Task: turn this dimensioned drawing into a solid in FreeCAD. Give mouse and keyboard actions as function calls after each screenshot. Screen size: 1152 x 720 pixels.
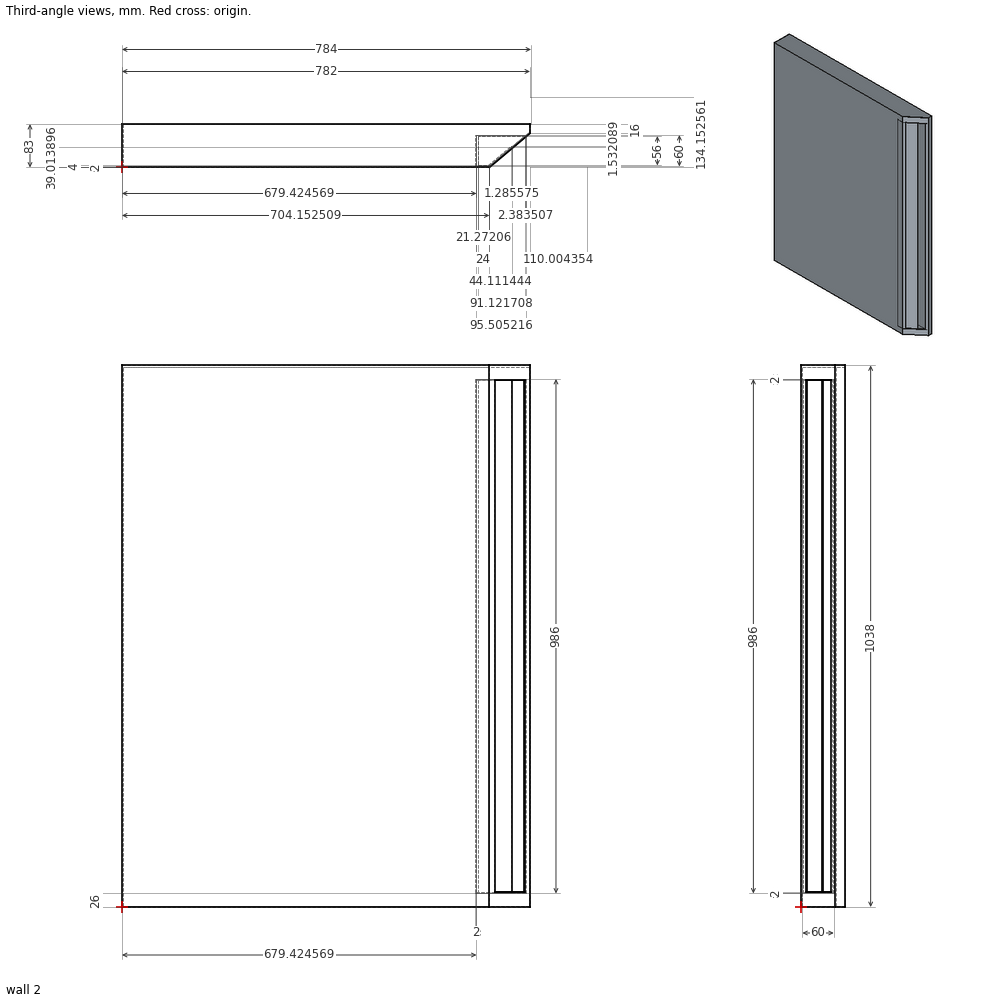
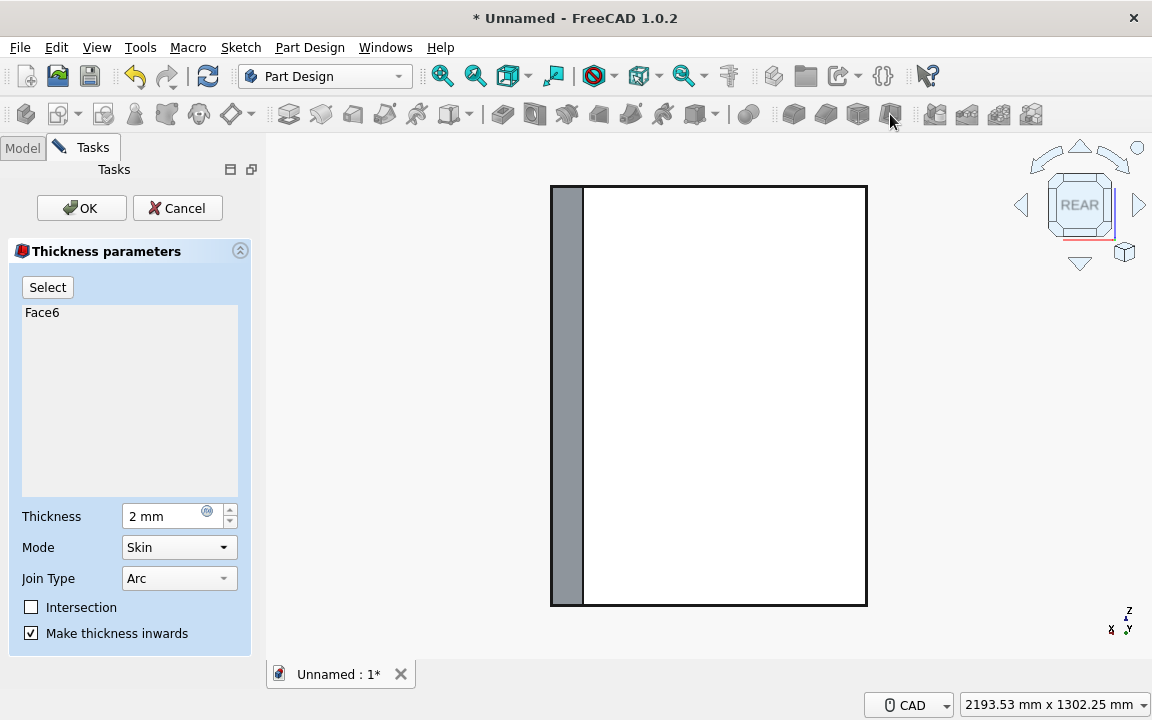
click(180, 578)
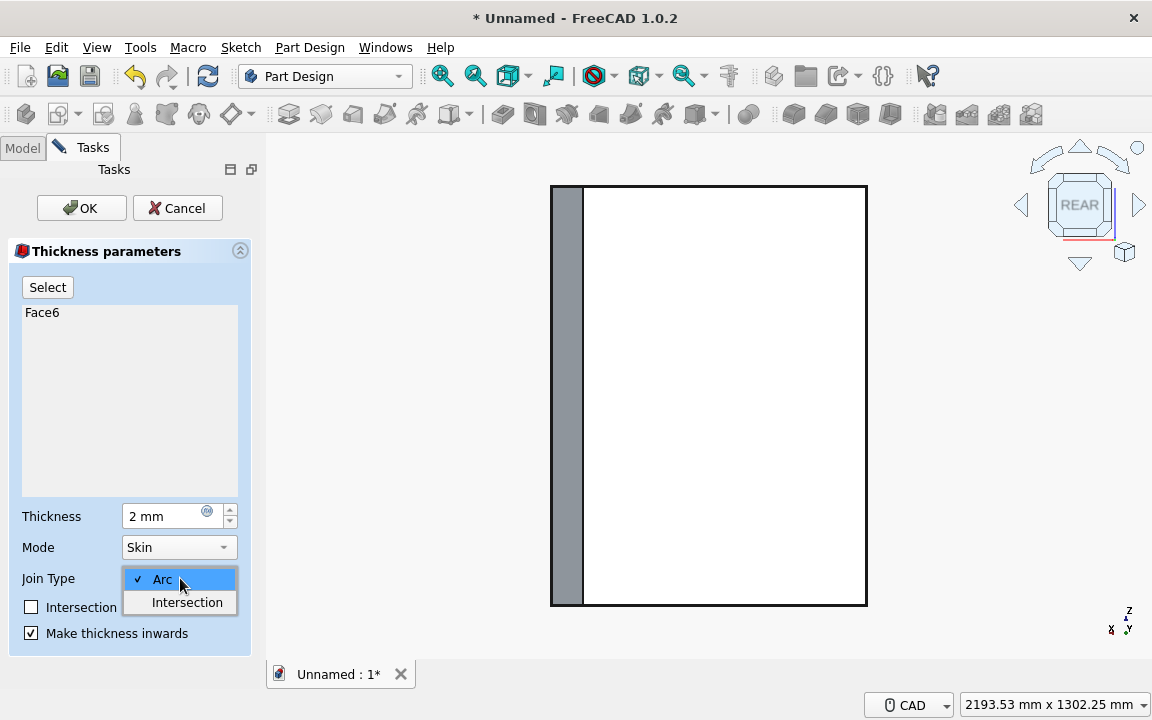
click(179, 602)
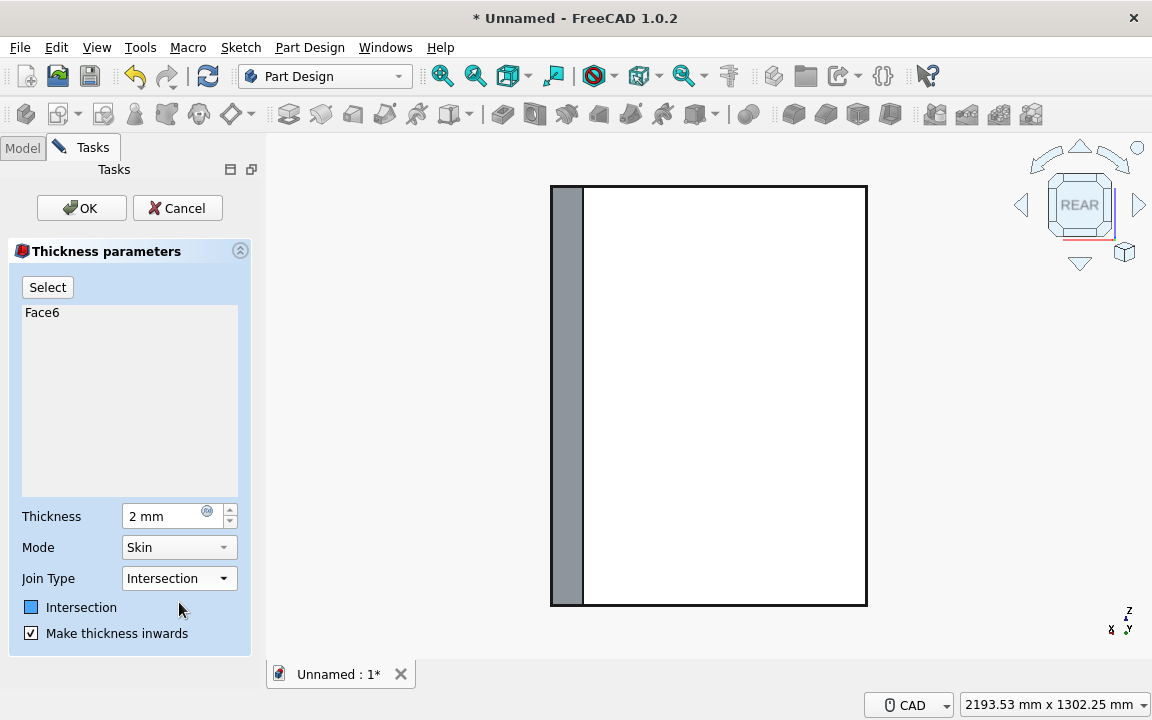
click(82, 208)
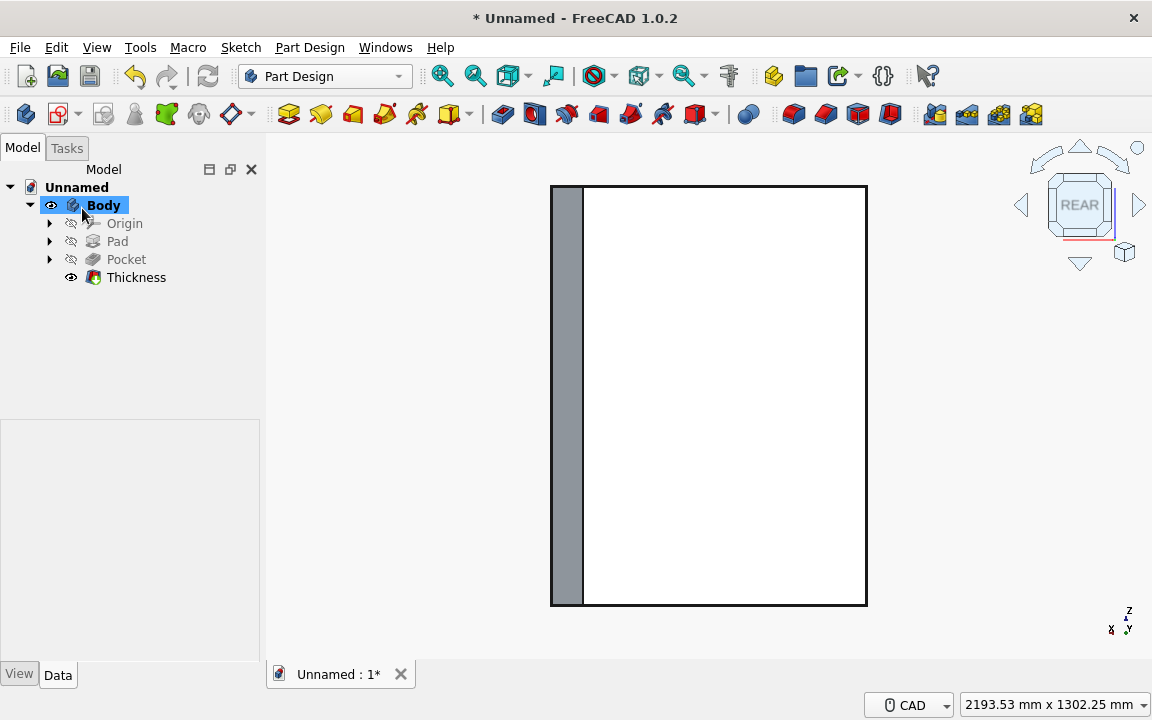
key(0)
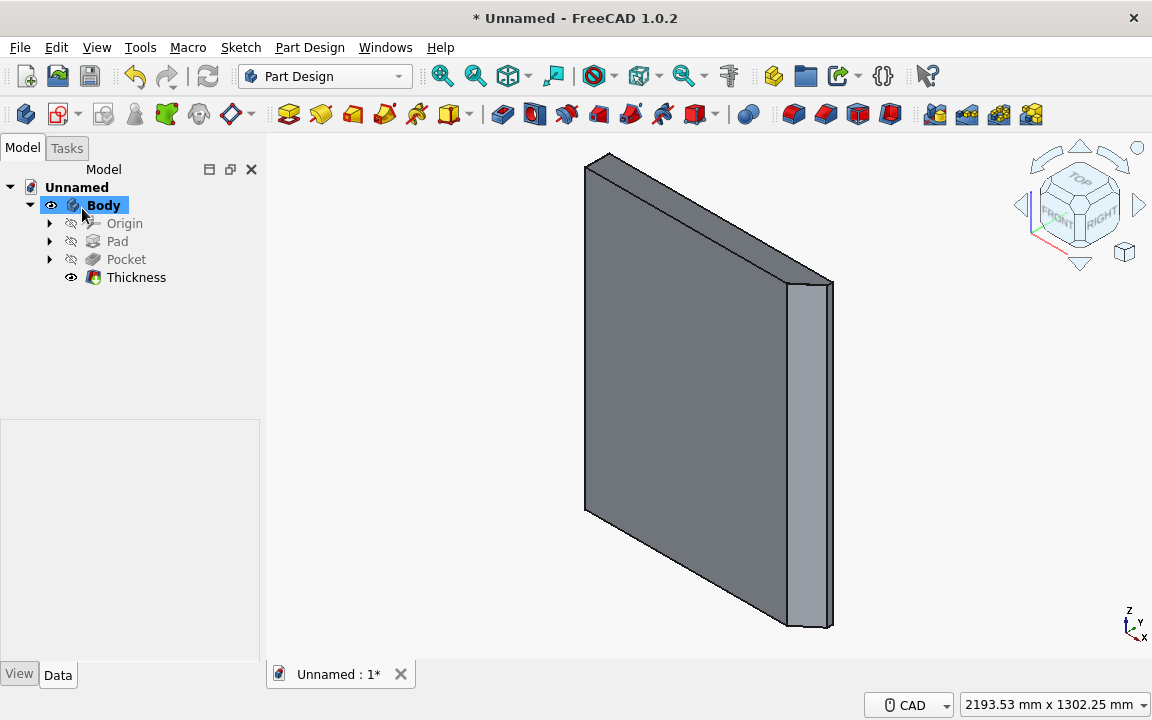
click(807, 308)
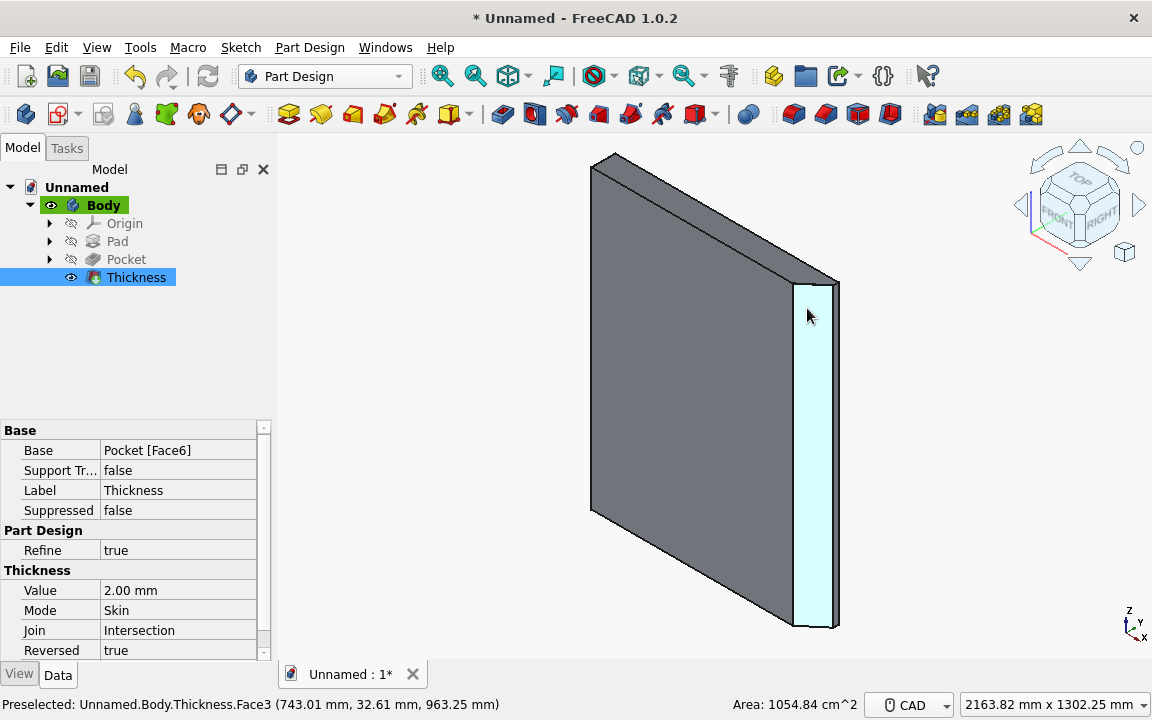
click(58, 114)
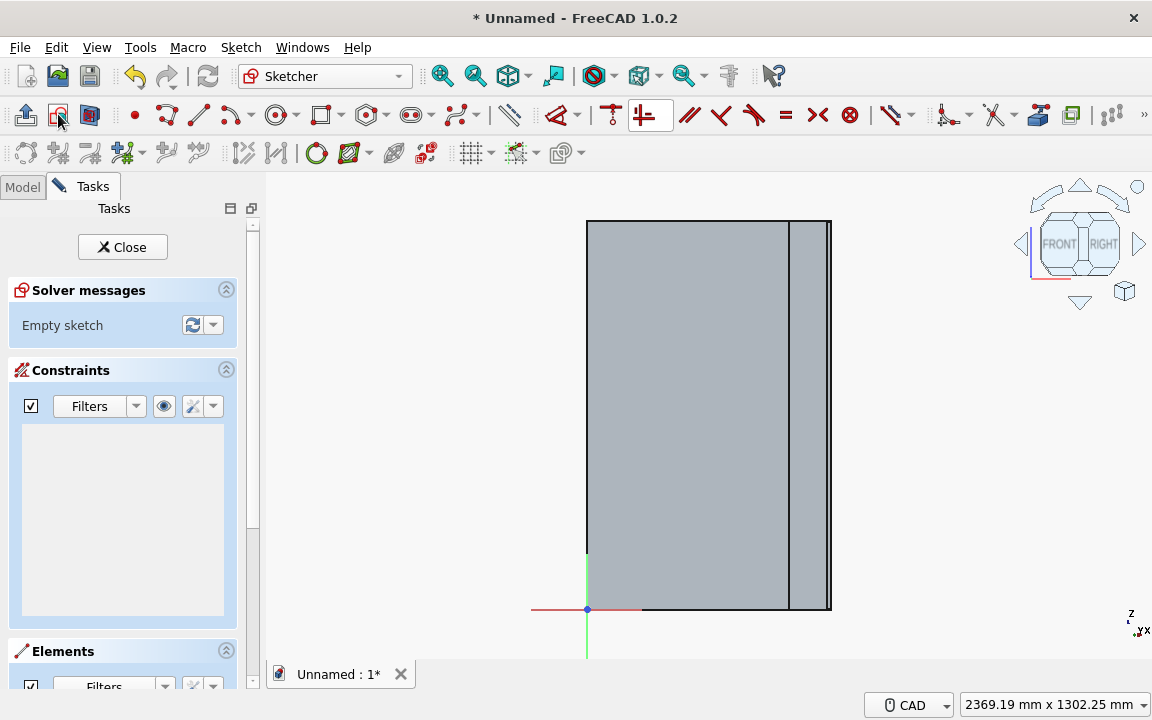
click(90, 116)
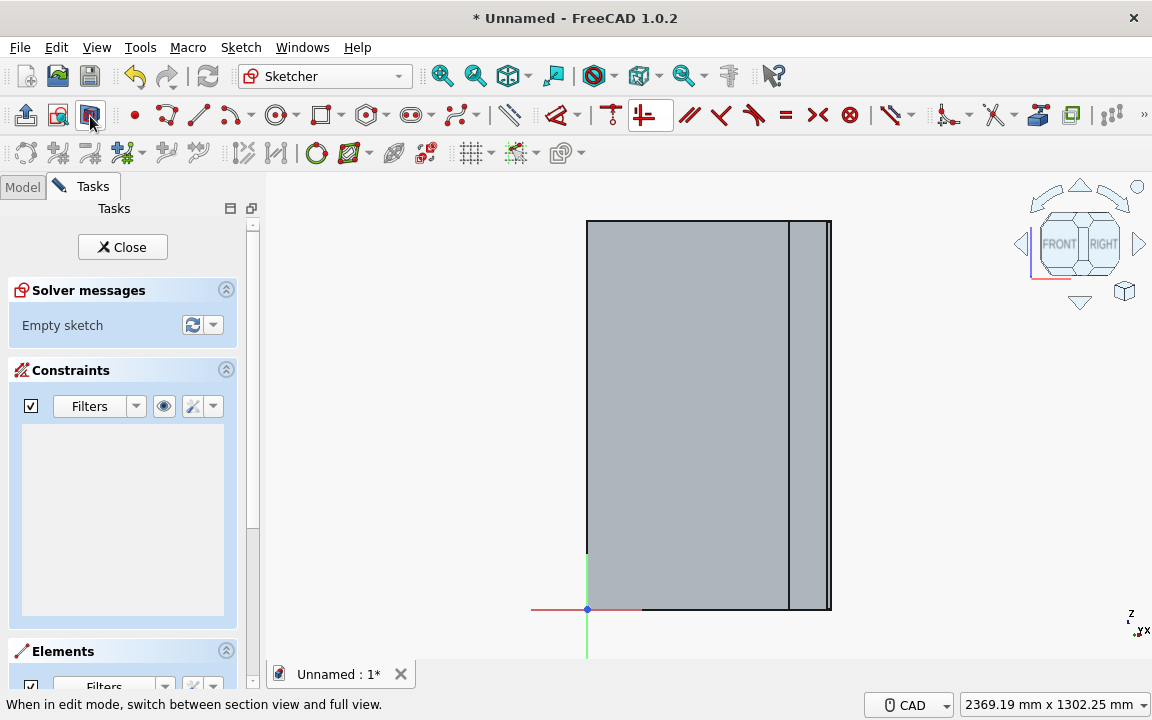
scroll(352, 392, down, 1)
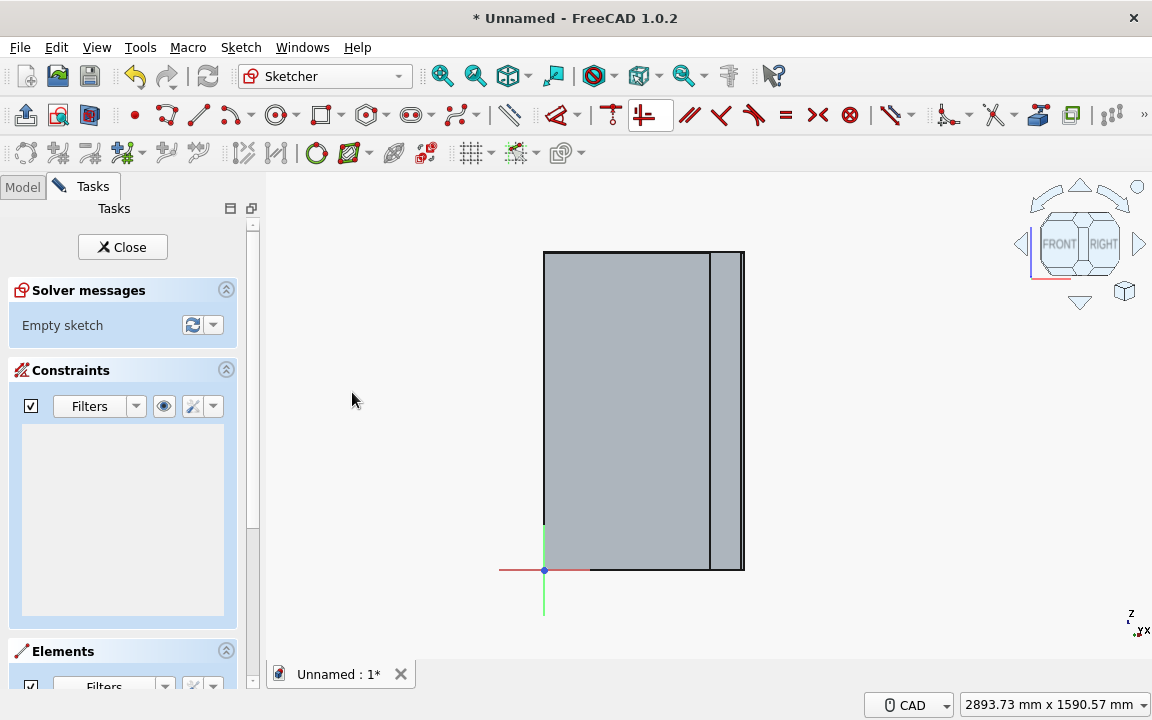
click(322, 116)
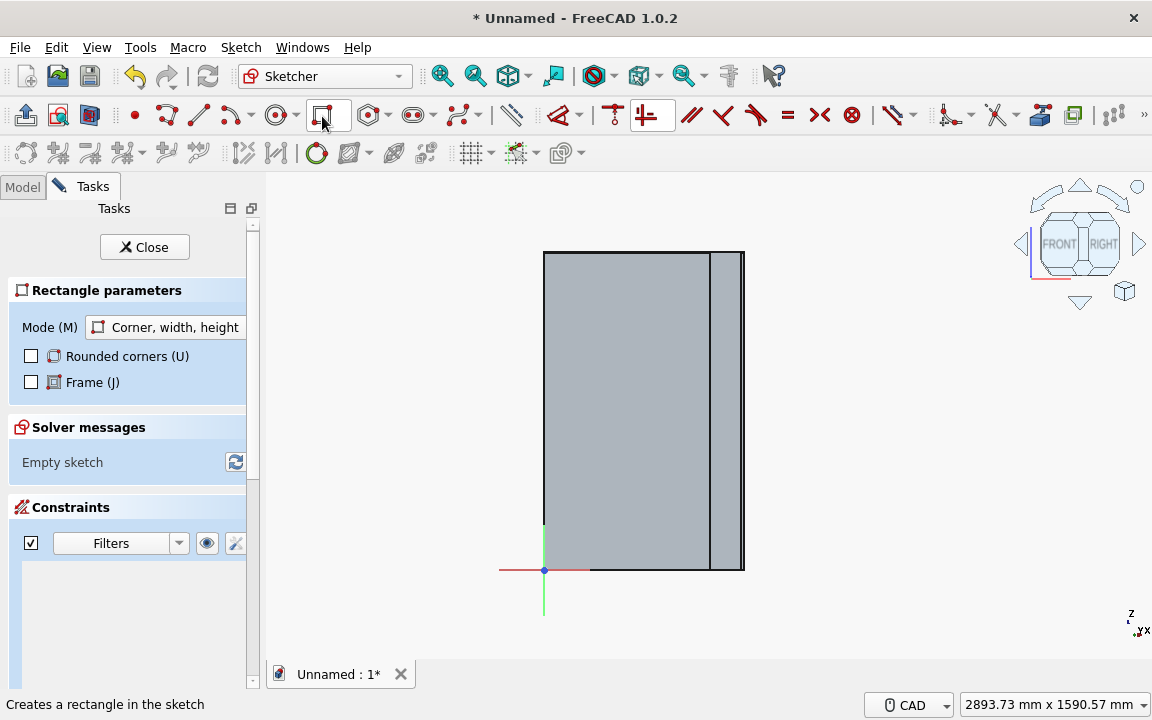
click(714, 261)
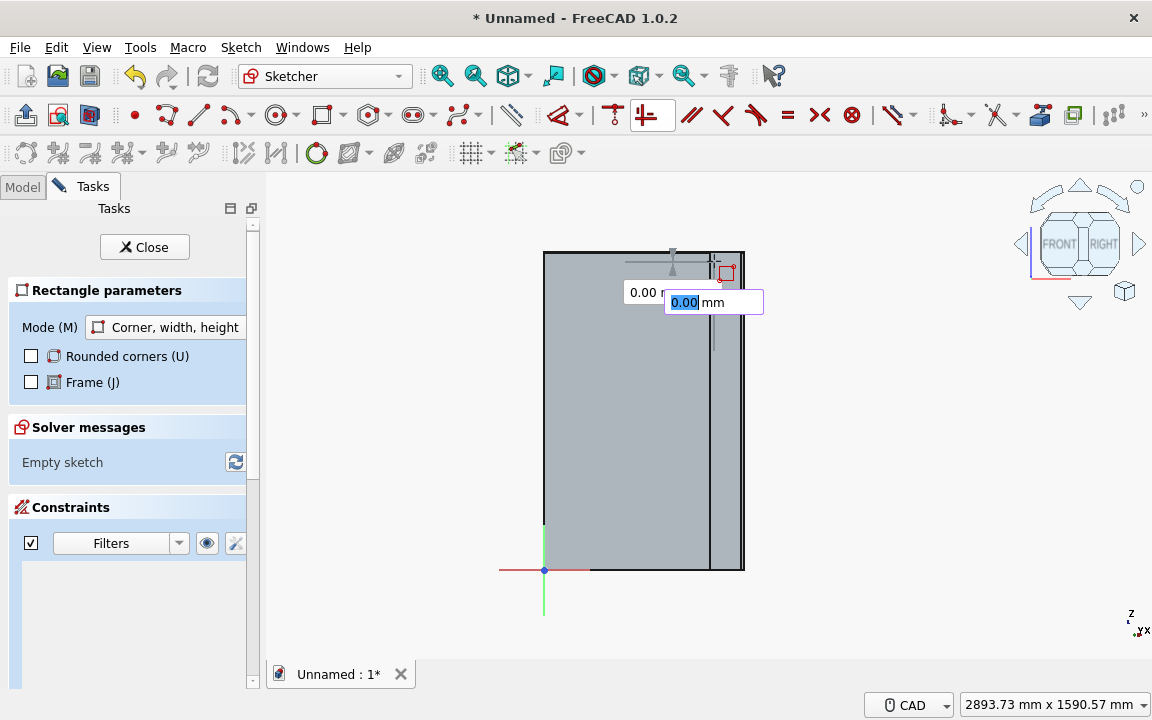
scroll(737, 562, up, 4)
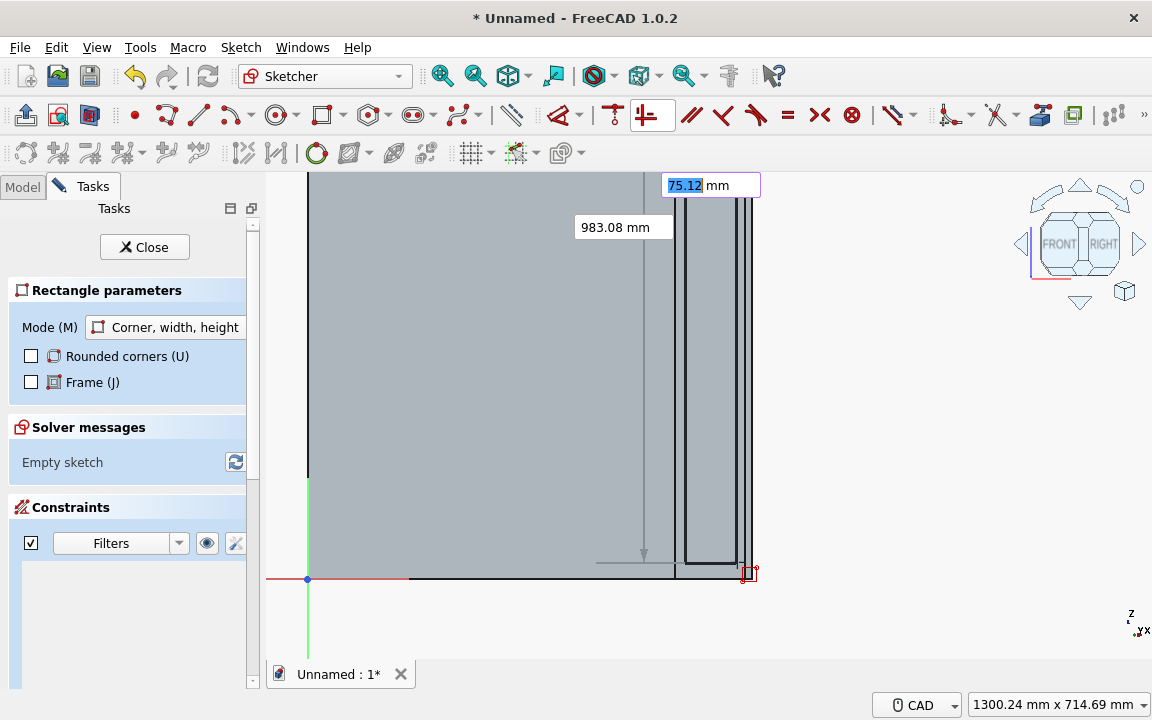
click(736, 560)
key(Escape)